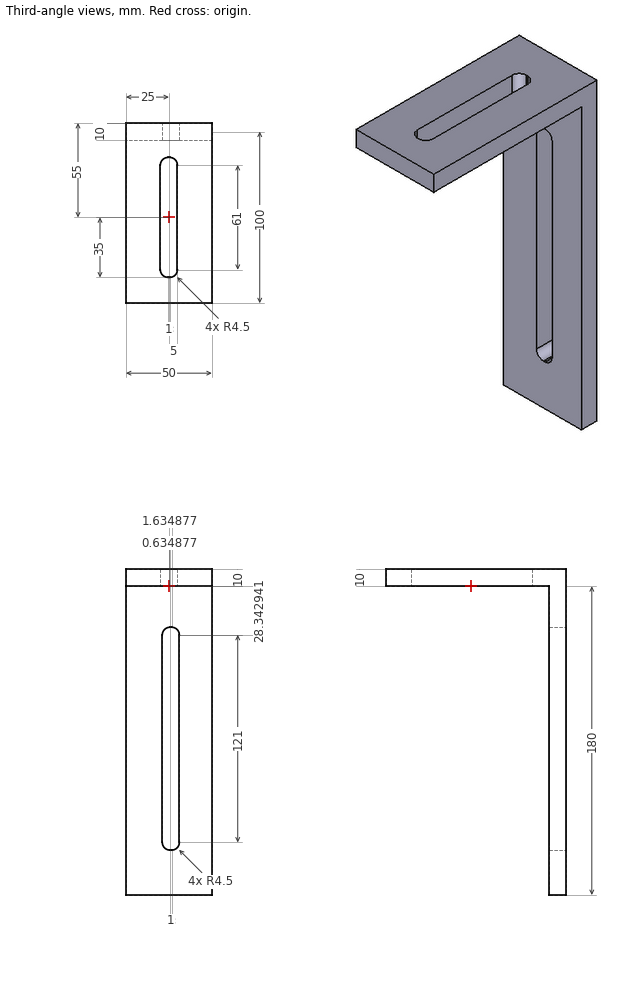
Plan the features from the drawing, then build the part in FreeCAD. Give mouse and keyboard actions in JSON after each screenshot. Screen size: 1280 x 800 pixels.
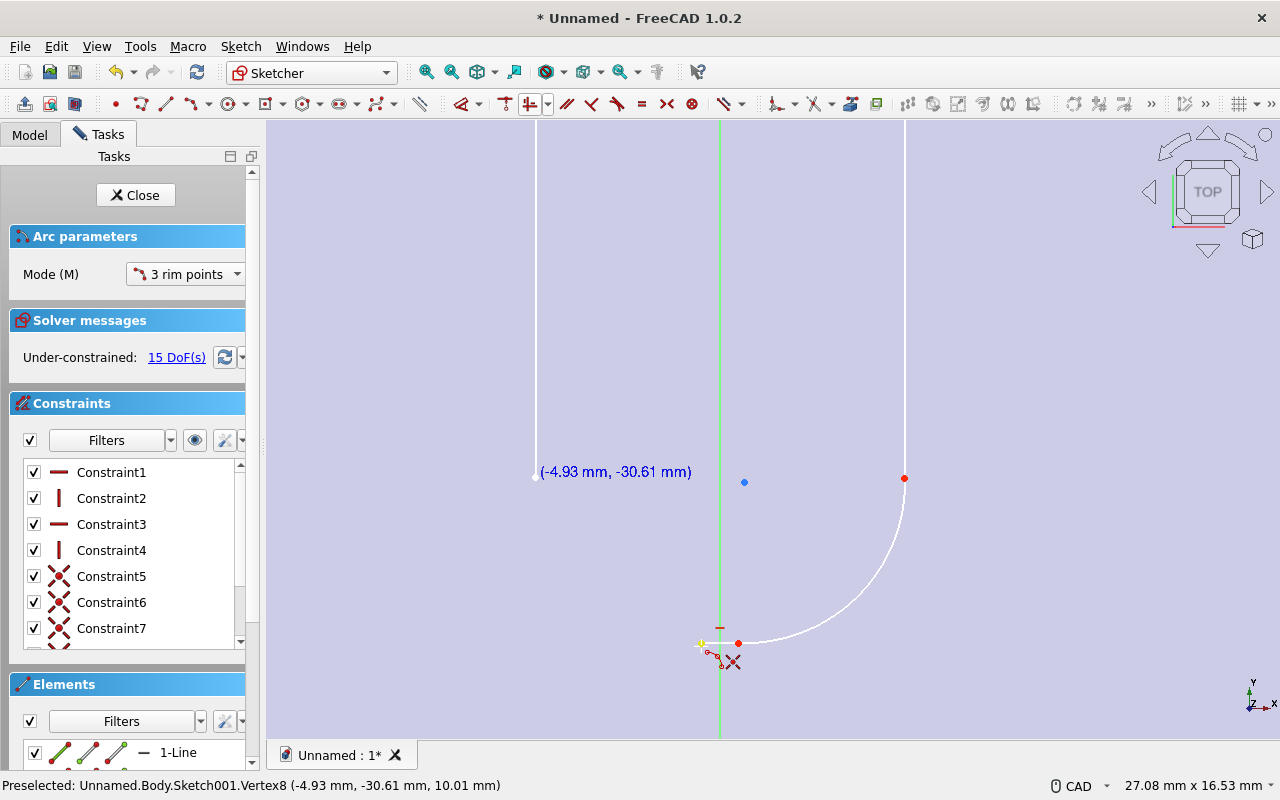
{"action": "left_click", "coordinate": [702, 643]}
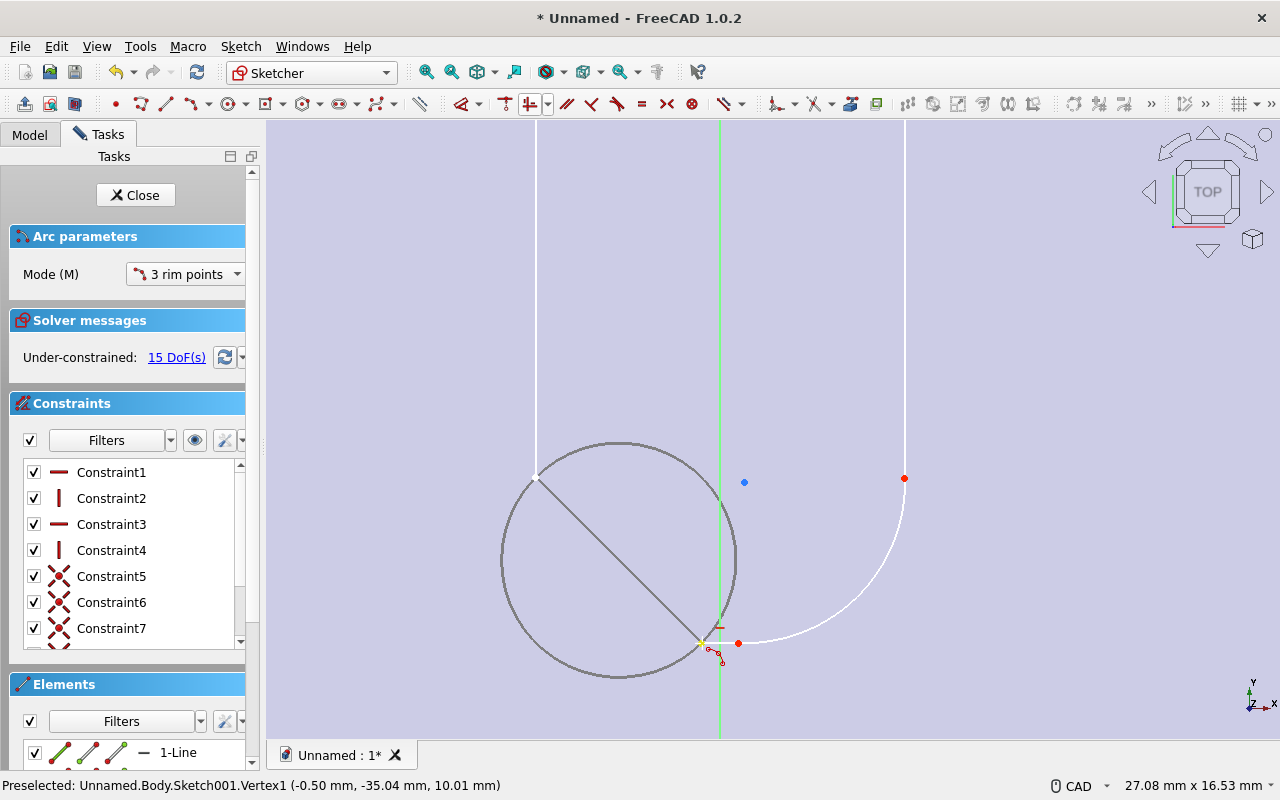
{"action": "scroll", "coordinate": [701, 647], "scroll_direction": "down", "scroll_amount": 9}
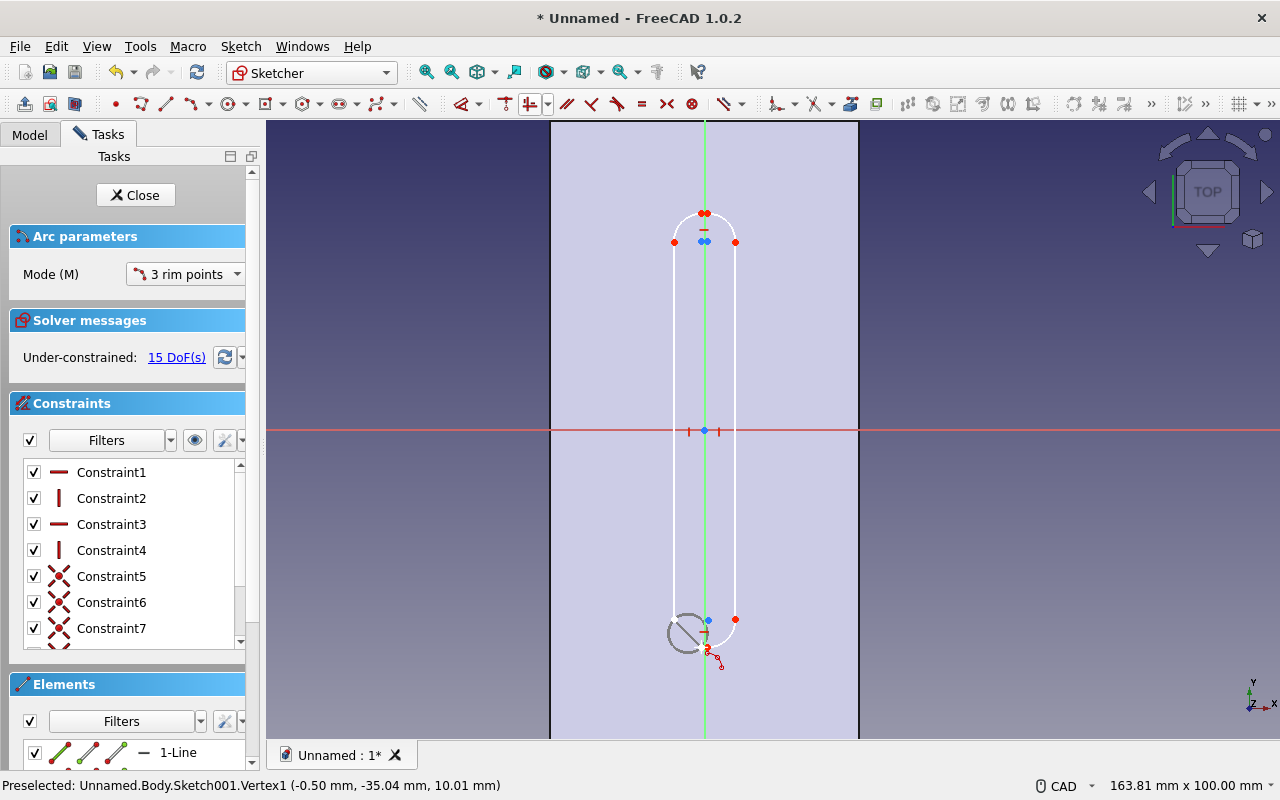
{"action": "scroll", "coordinate": [682, 639], "scroll_direction": "up", "scroll_amount": 4}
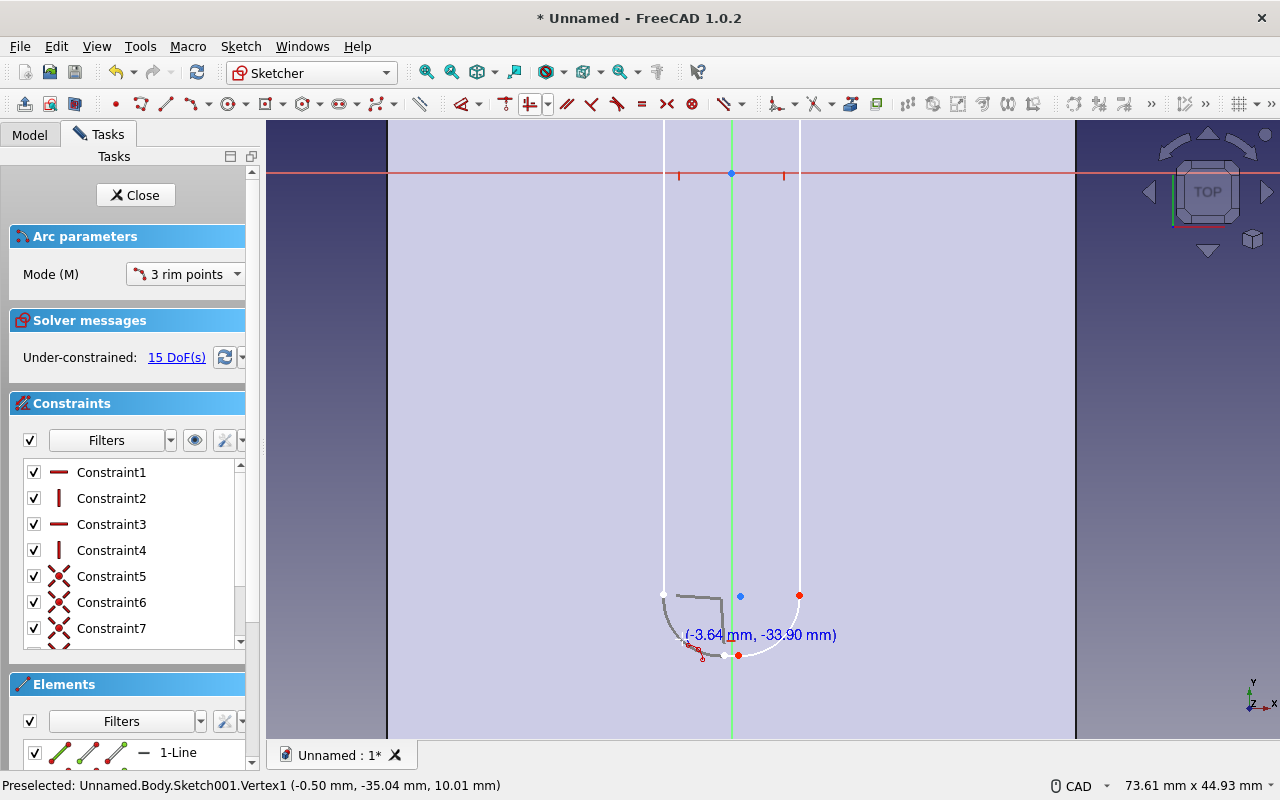
{"action": "left_click", "coordinate": [681, 637]}
{"action": "key", "text": "Escape"}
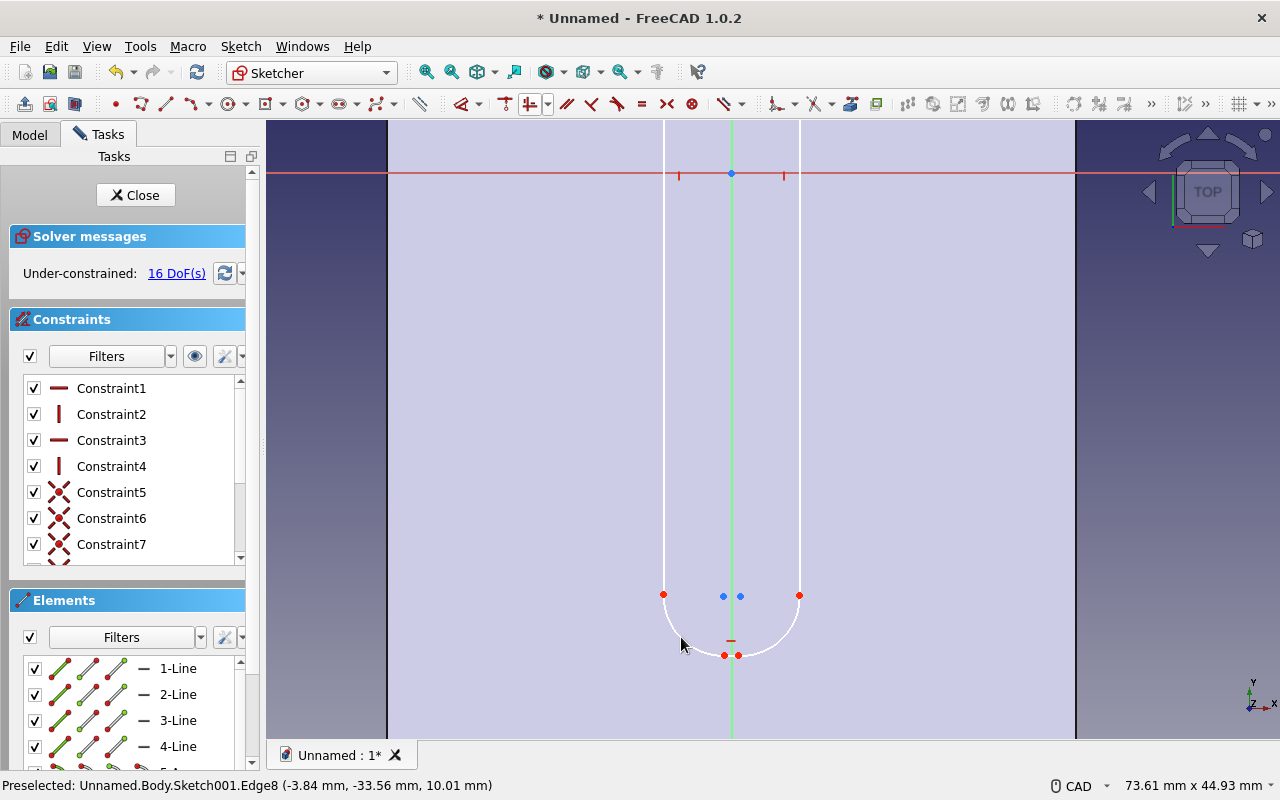
{"action": "scroll", "coordinate": [732, 656], "scroll_direction": "up", "scroll_amount": 4}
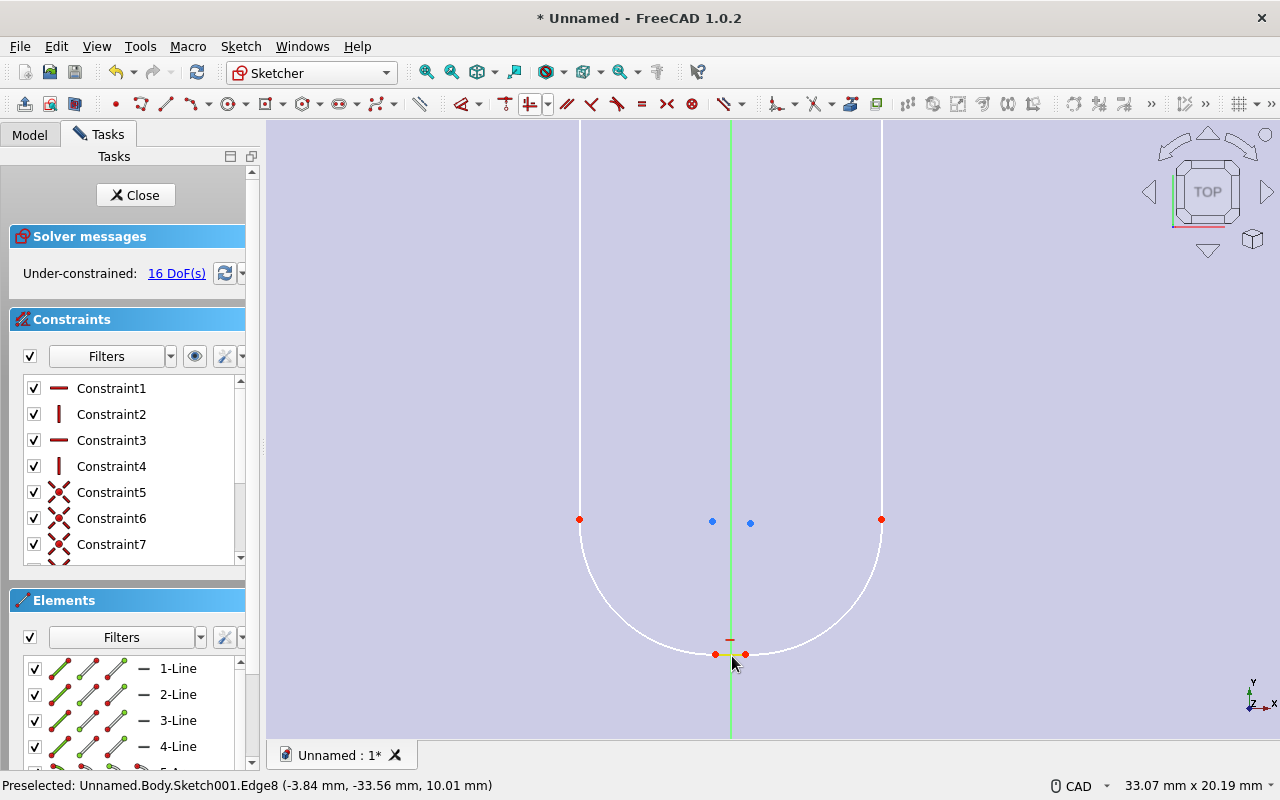
{"action": "left_click", "coordinate": [731, 655]}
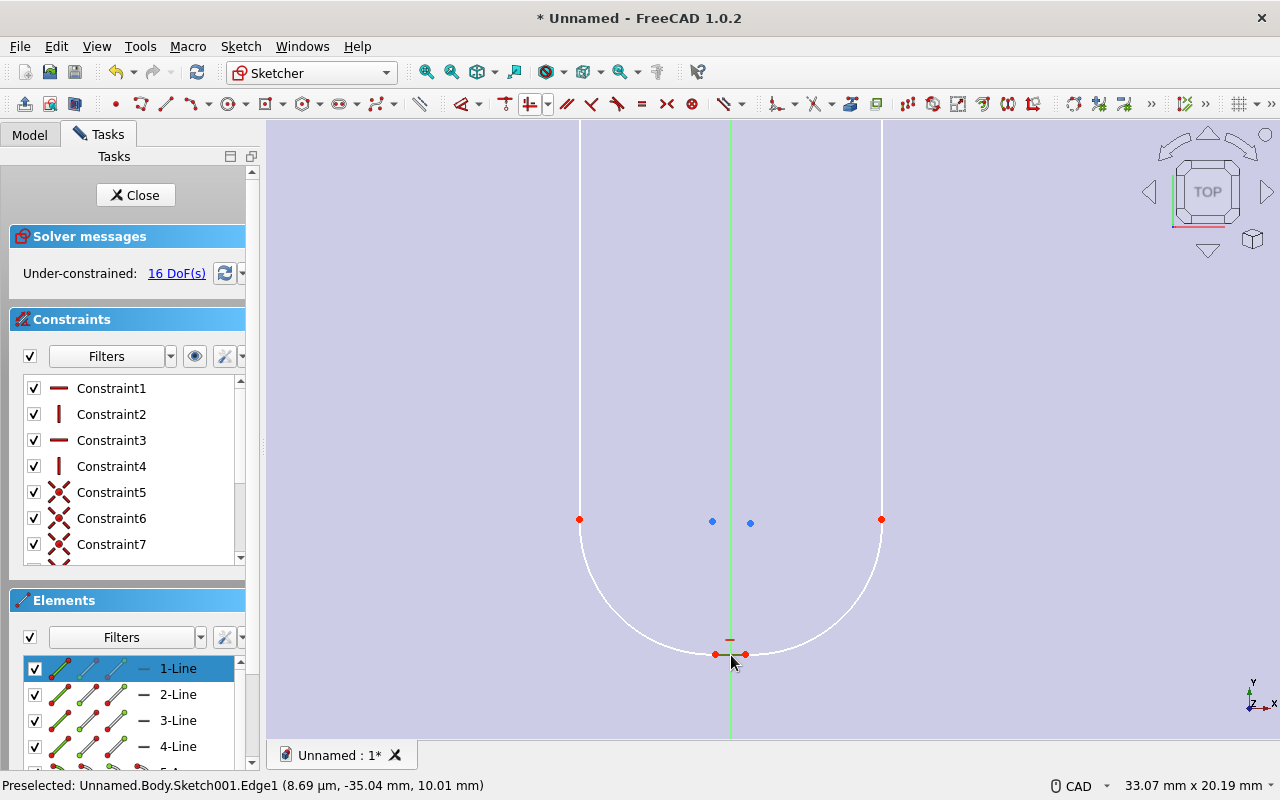
{"action": "scroll", "coordinate": [698, 644], "scroll_direction": "down", "scroll_amount": 8}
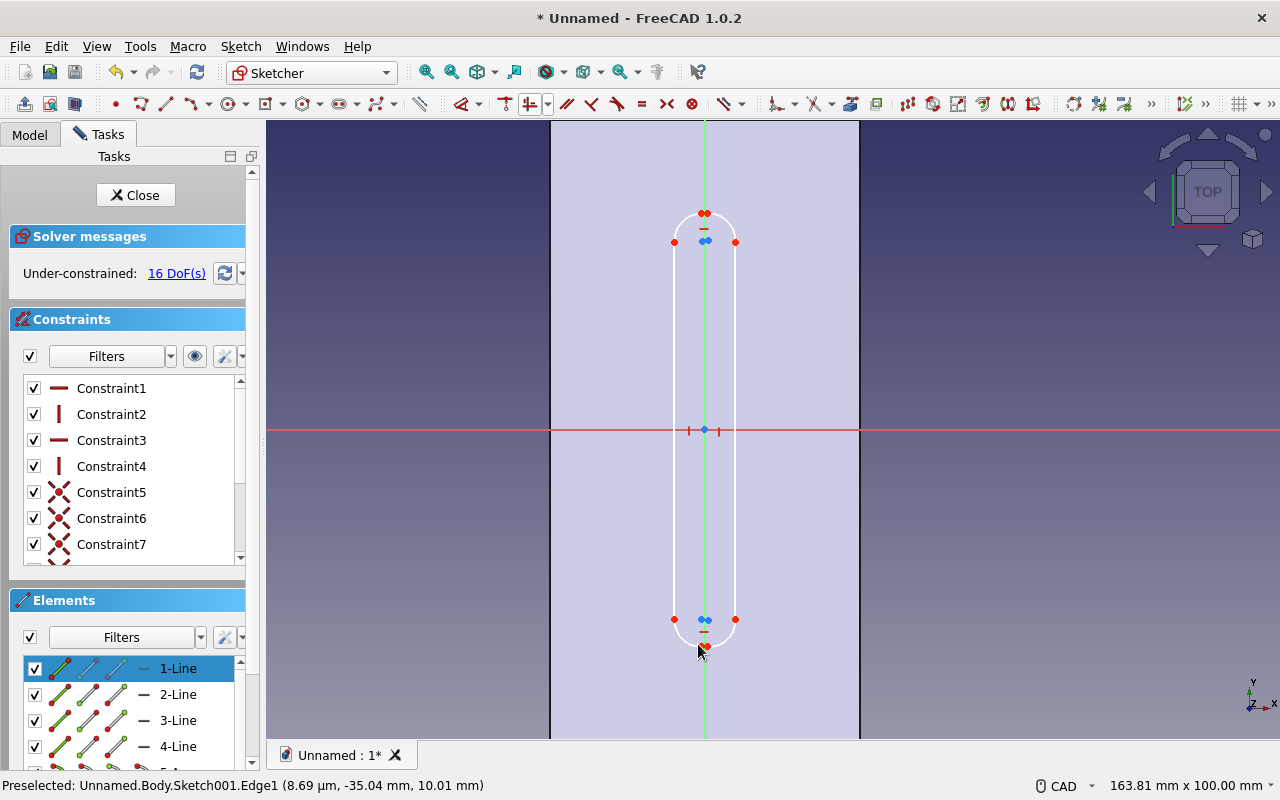
{"action": "left_click", "coordinate": [721, 644]}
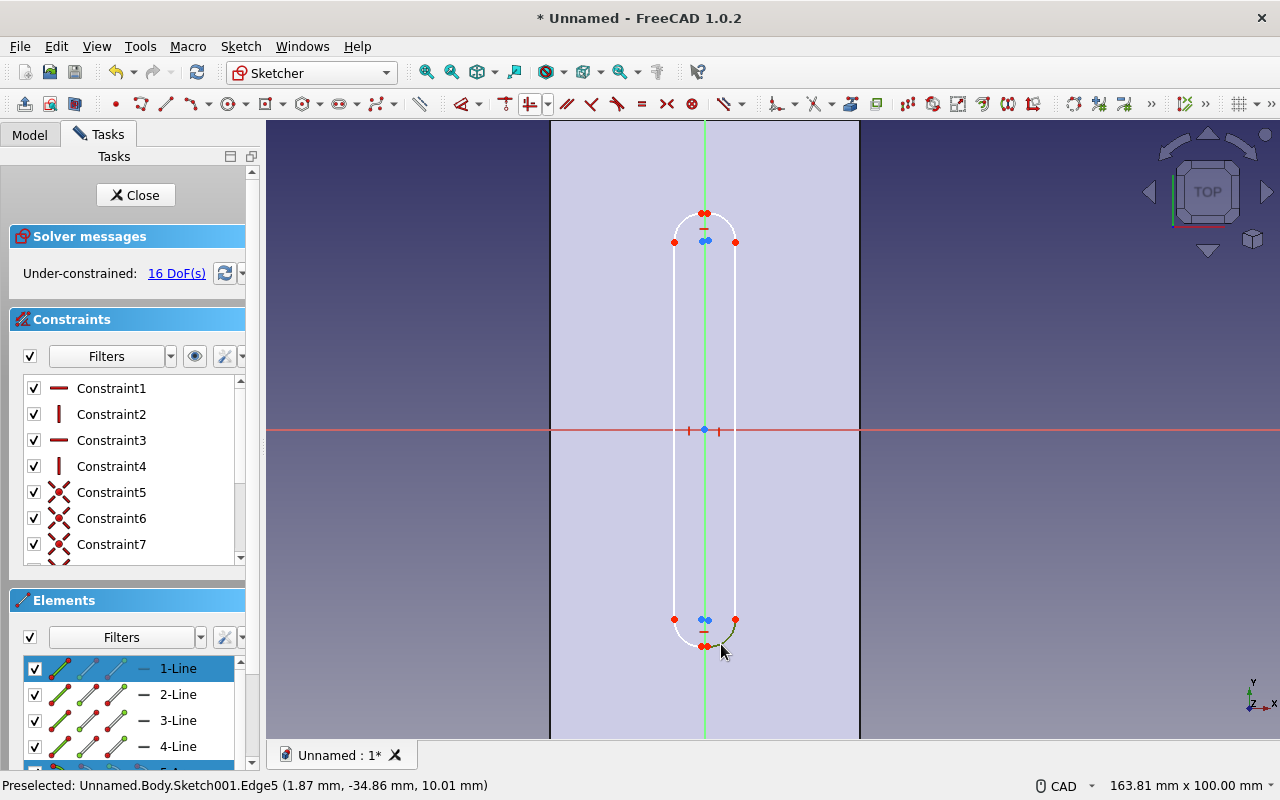
{"action": "left_click", "coordinate": [617, 104]}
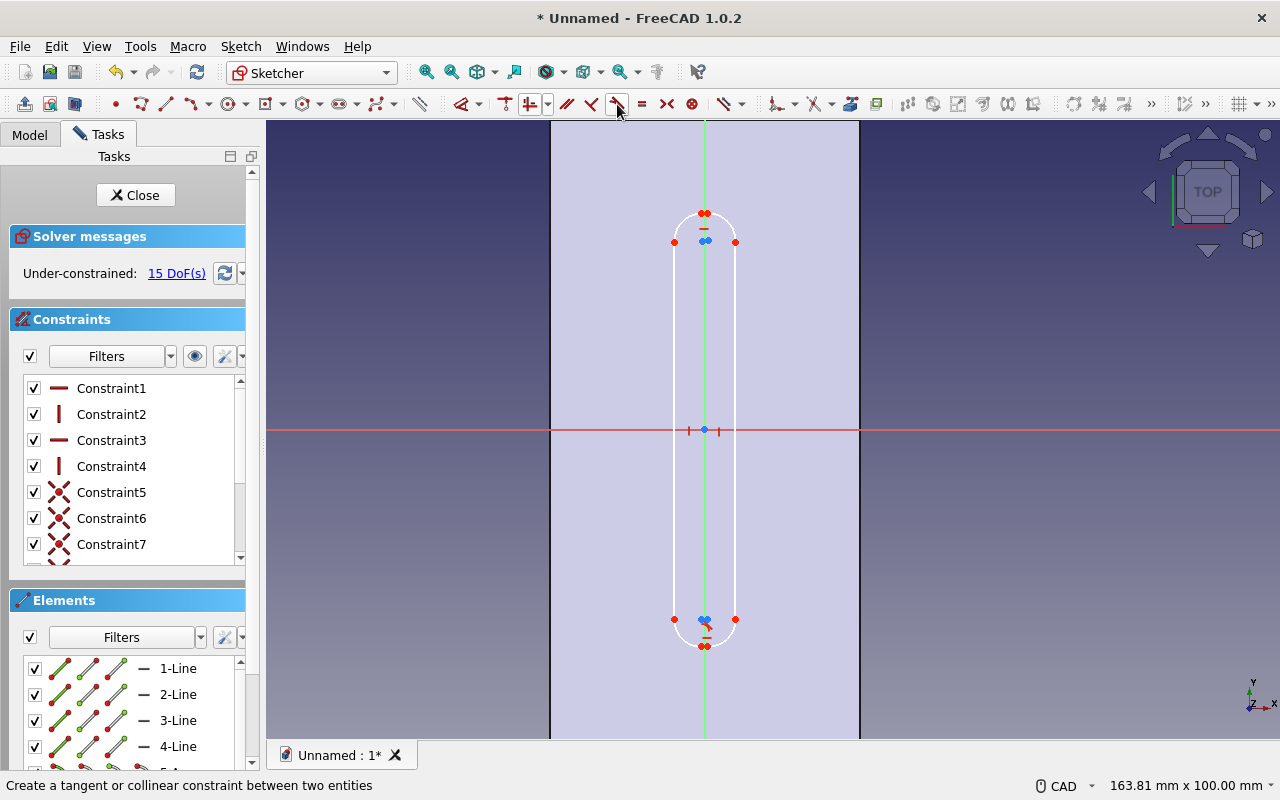
{"action": "scroll", "coordinate": [705, 647], "scroll_direction": "up", "scroll_amount": 8}